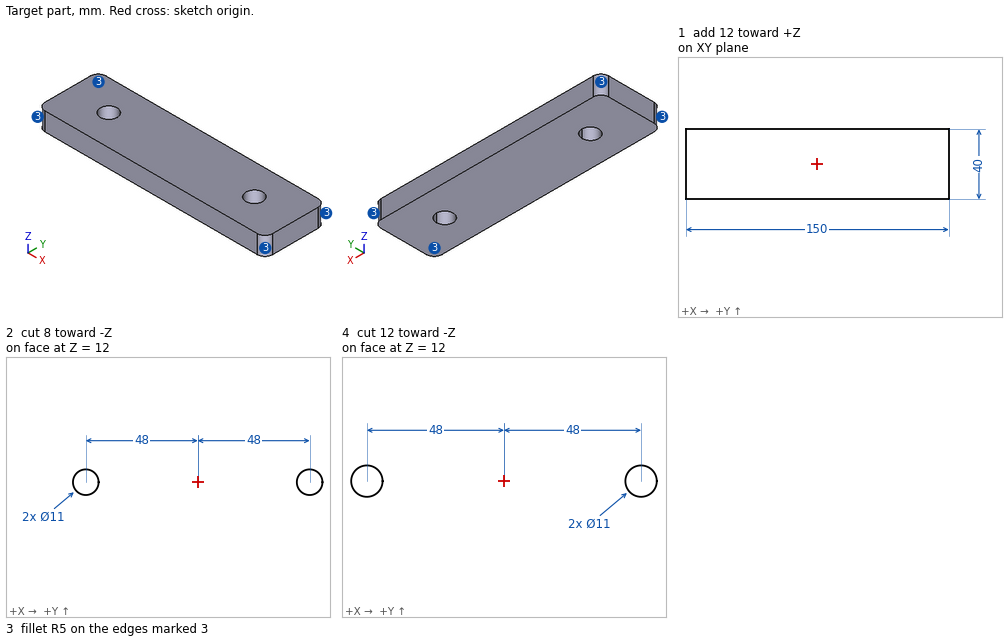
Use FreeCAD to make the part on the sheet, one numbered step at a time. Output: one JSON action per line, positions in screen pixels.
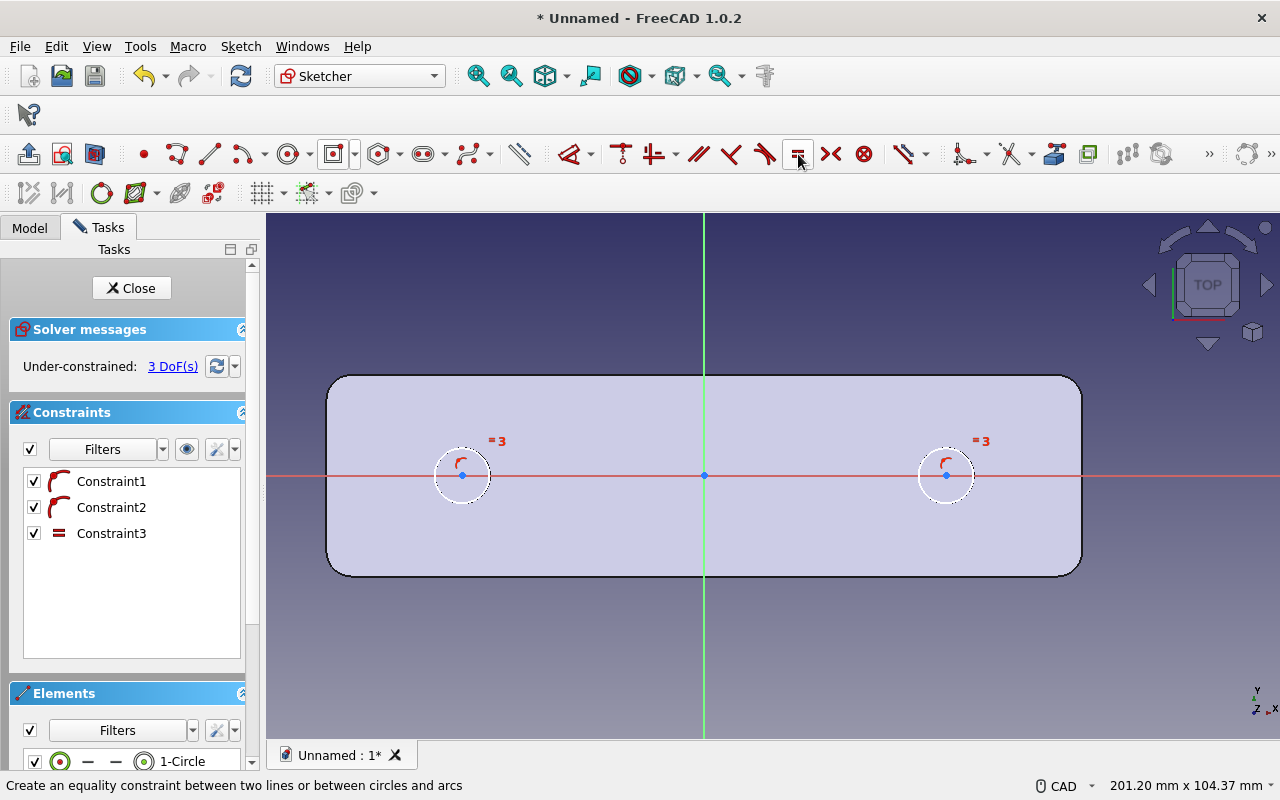
{"action": "left_click", "coordinate": [568, 154]}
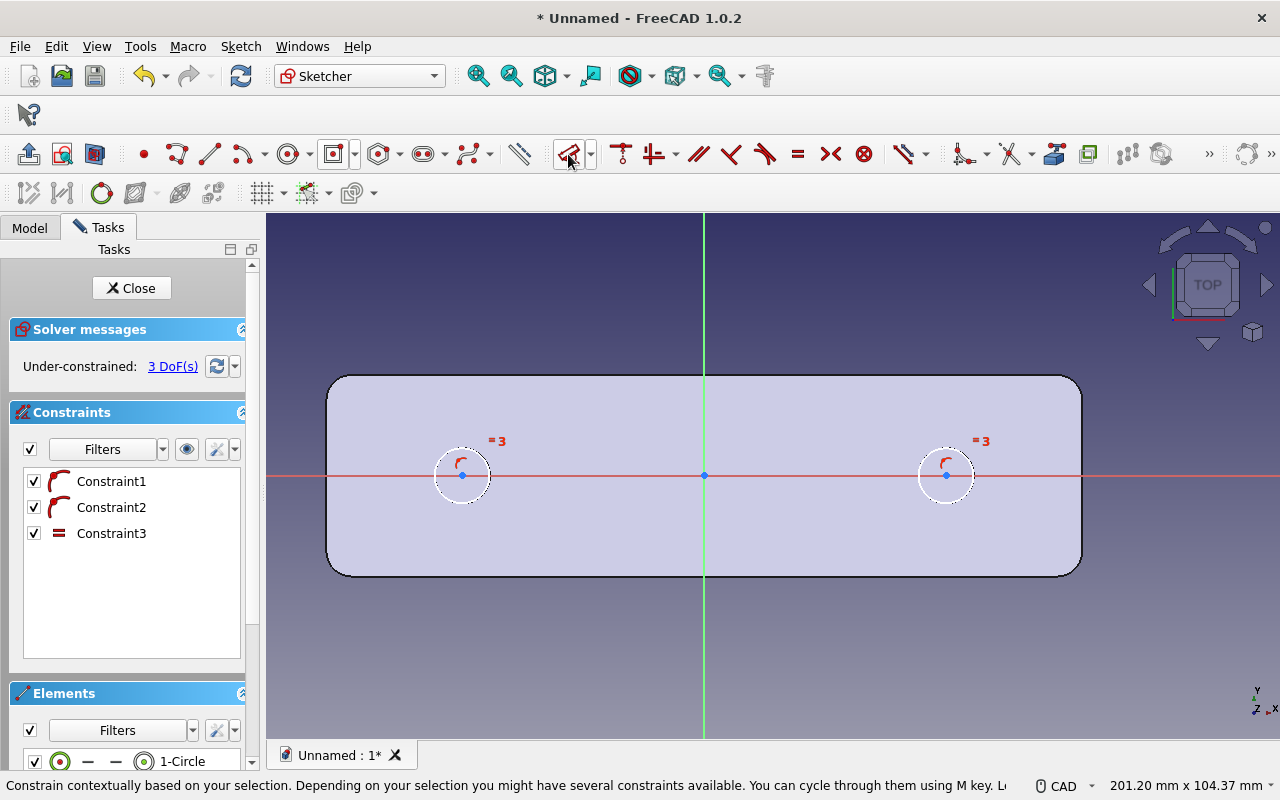
{"action": "left_click", "coordinate": [965, 456]}
{"action": "left_click", "coordinate": [987, 433]}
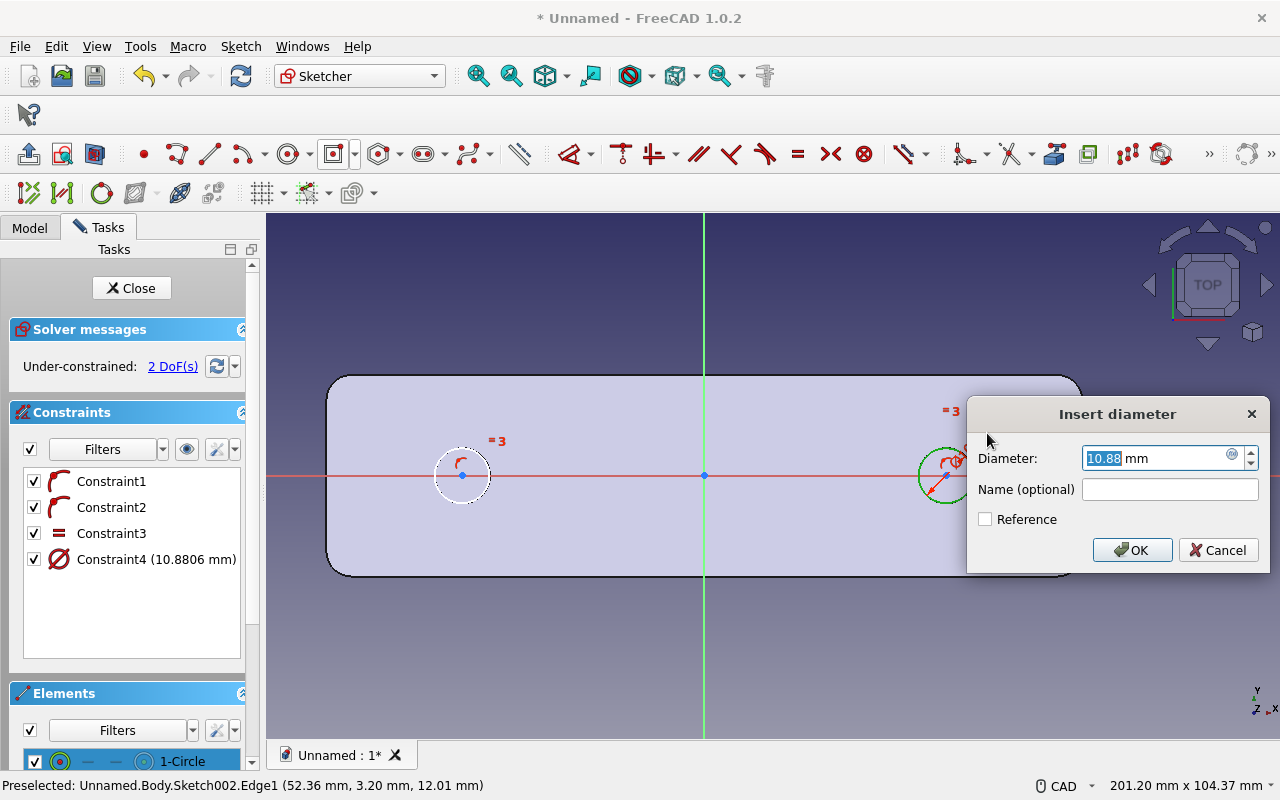
{"action": "type", "text": "11"}
{"action": "key", "text": "Return"}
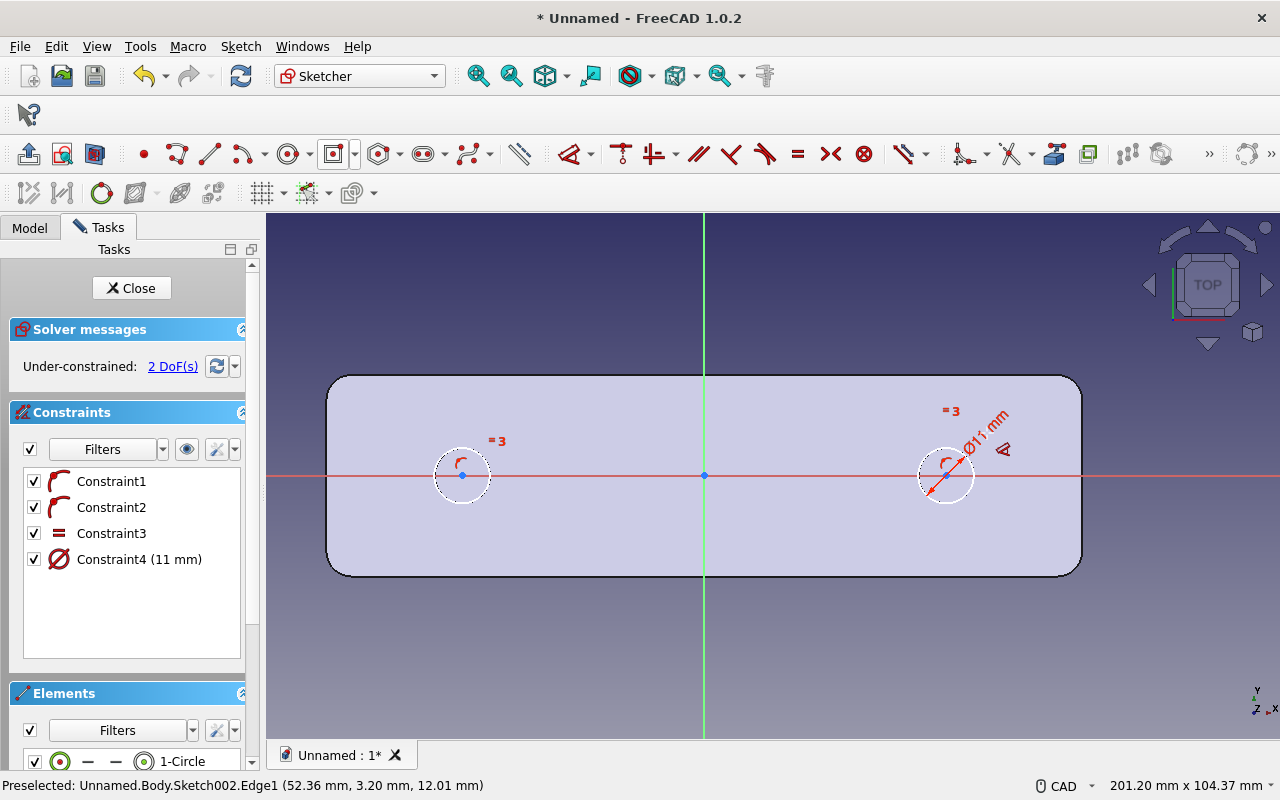
{"action": "left_click", "coordinate": [946, 476]}
{"action": "left_click", "coordinate": [825, 510]}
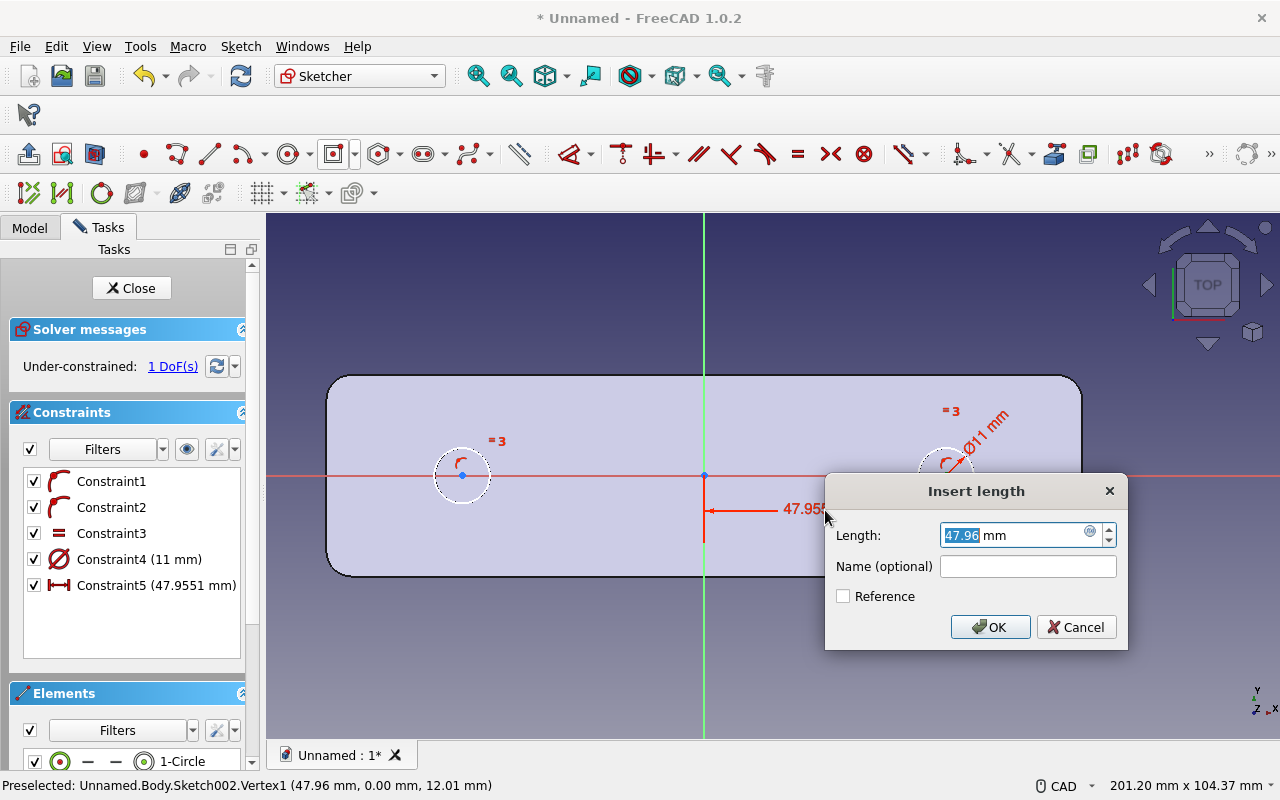
{"action": "type", "text": "48"}
{"action": "key", "text": "Return"}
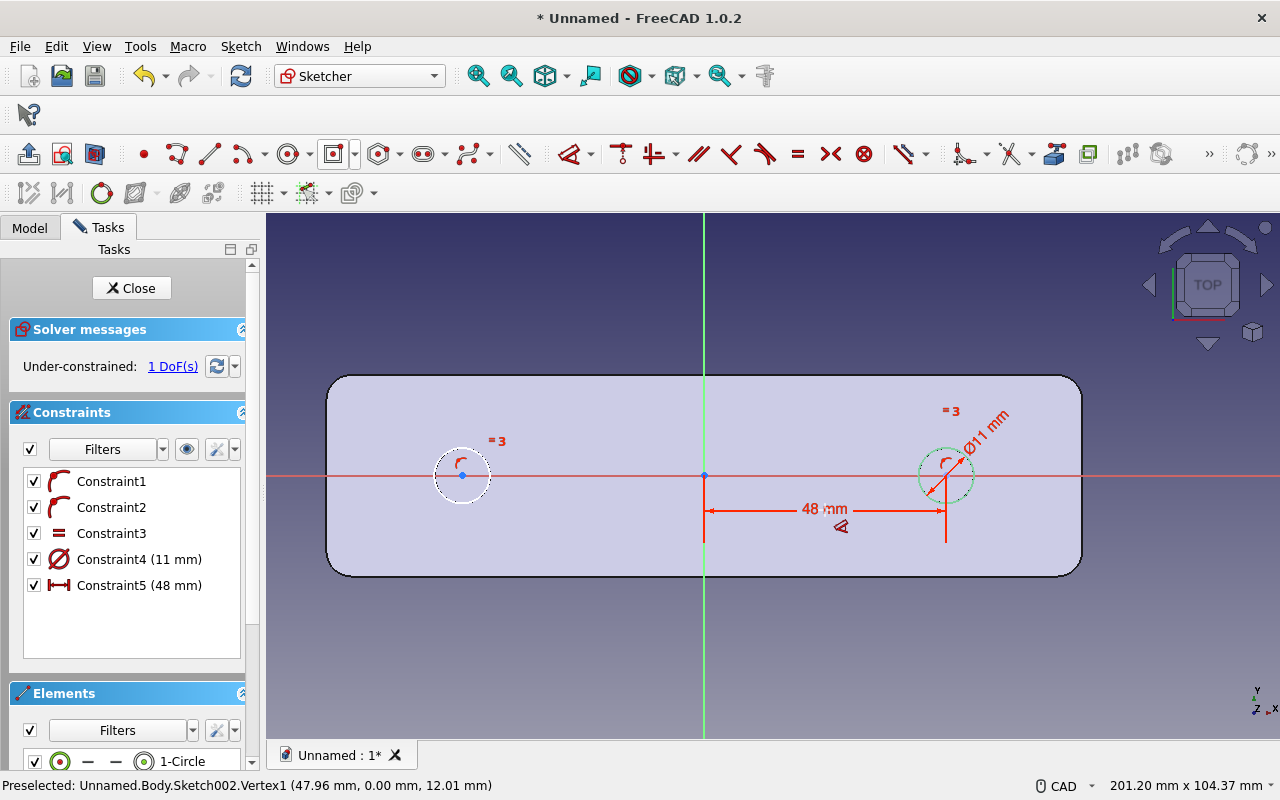
{"action": "left_click", "coordinate": [462, 476]}
{"action": "left_click", "coordinate": [583, 510]}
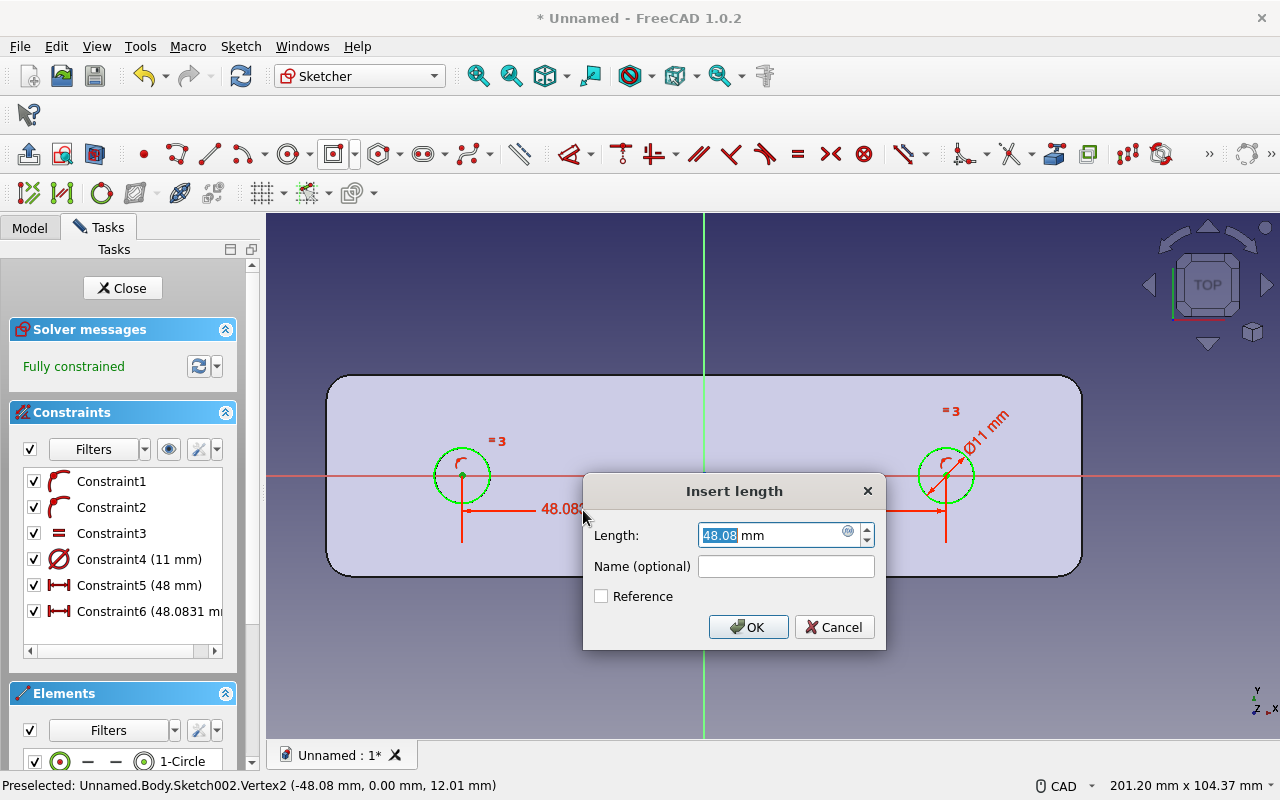
{"action": "type", "text": "48"}
{"action": "key", "text": "Return"}
{"action": "key", "text": "Escape"}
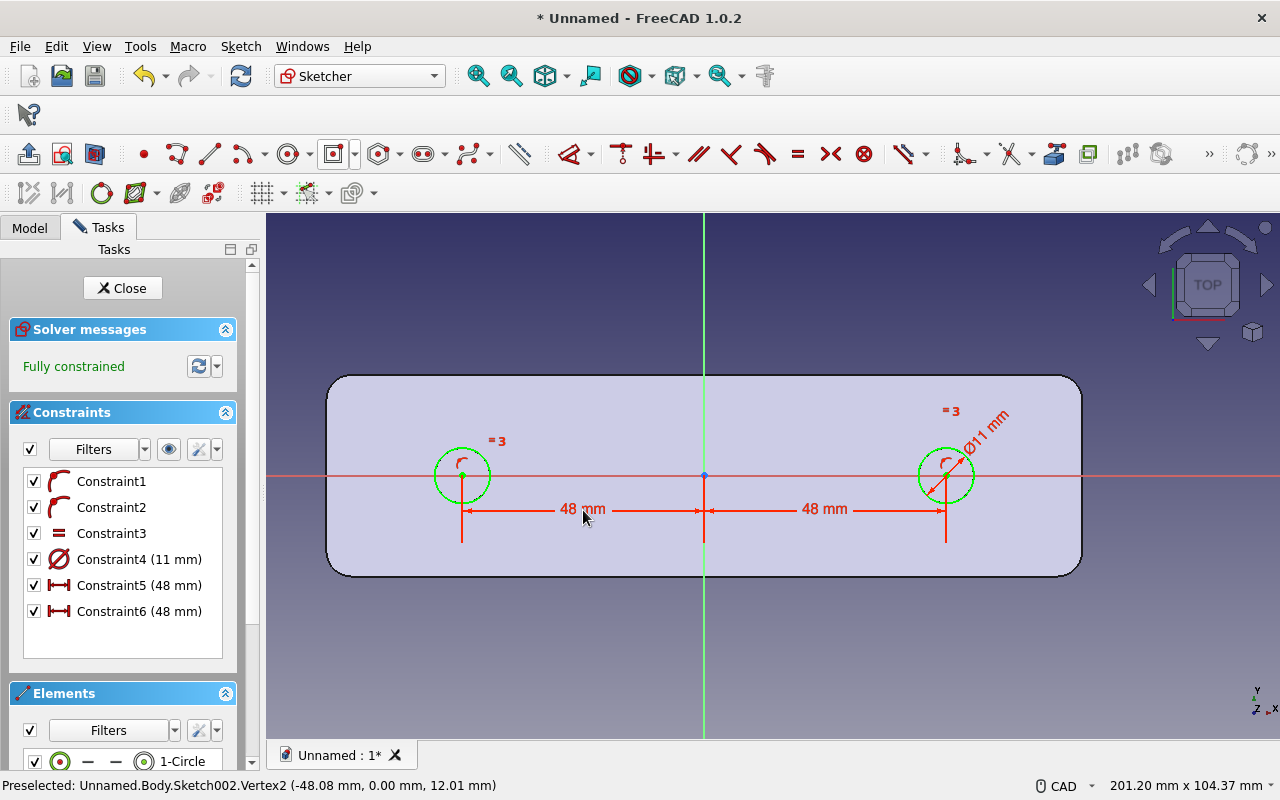
{"action": "left_click", "coordinate": [123, 288]}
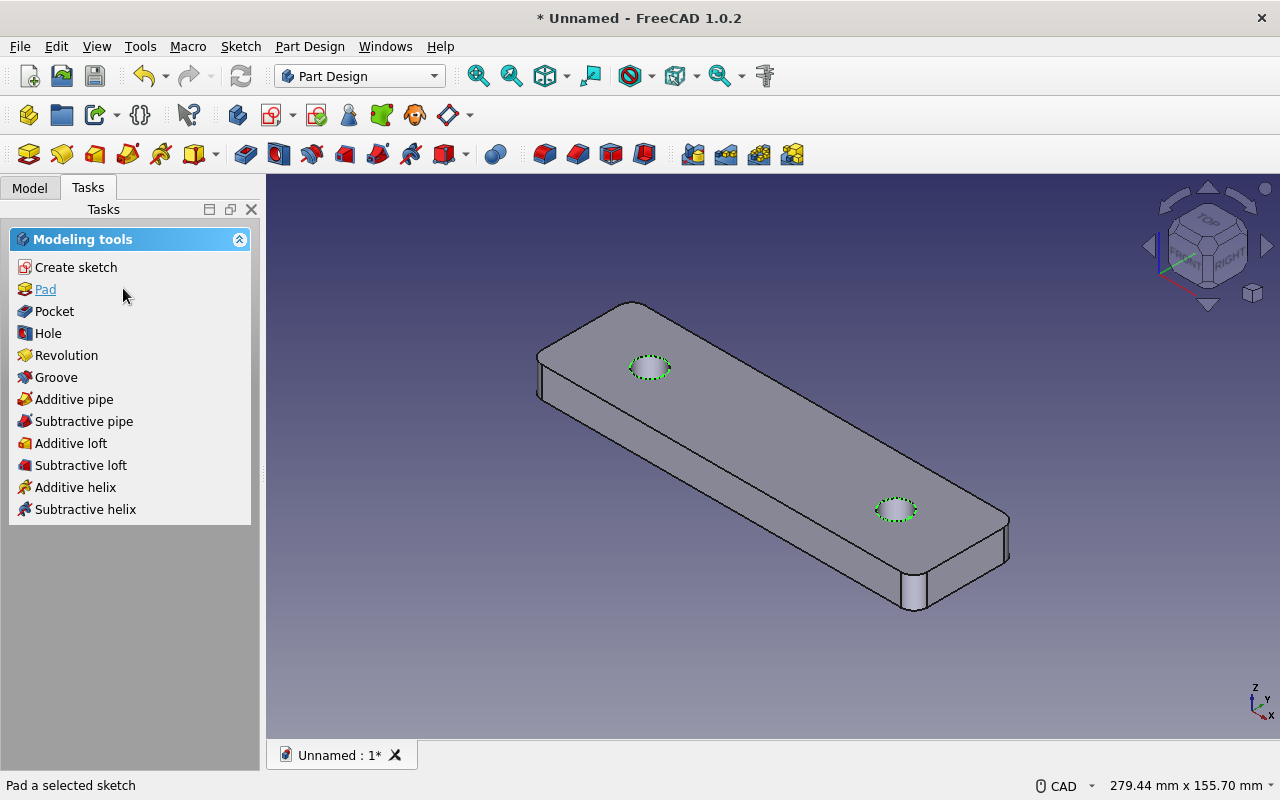
{"action": "left_click", "coordinate": [246, 154]}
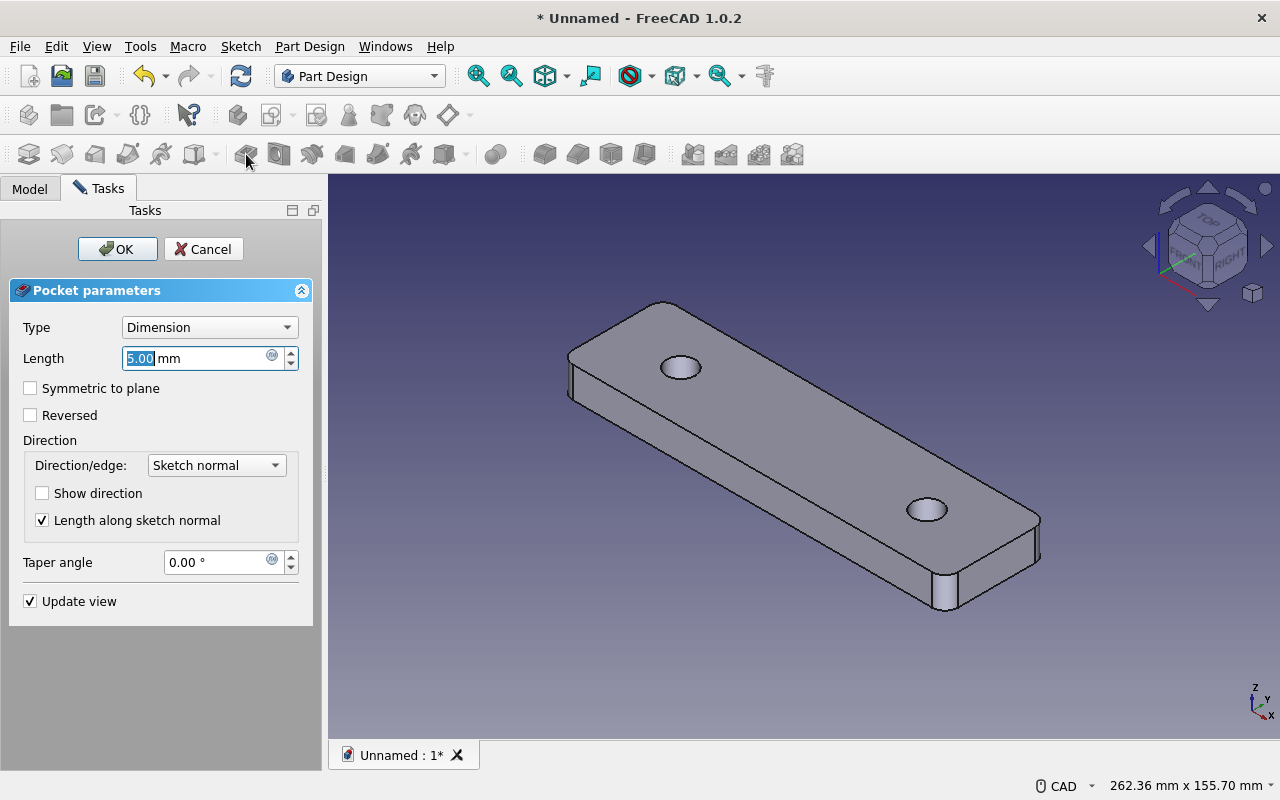
{"action": "type", "text": "12"}
{"action": "key", "text": "Tab"}